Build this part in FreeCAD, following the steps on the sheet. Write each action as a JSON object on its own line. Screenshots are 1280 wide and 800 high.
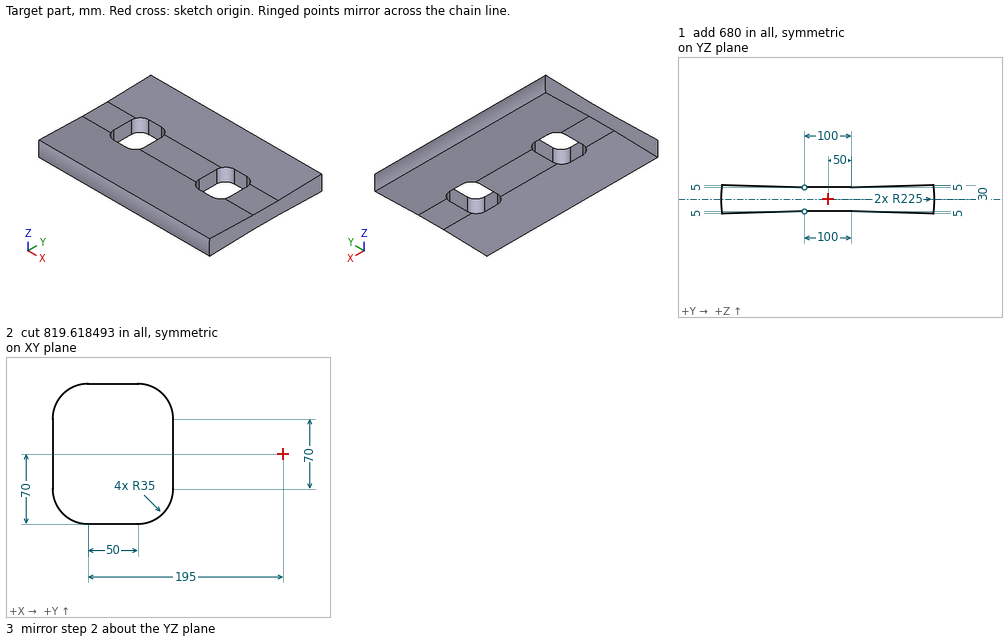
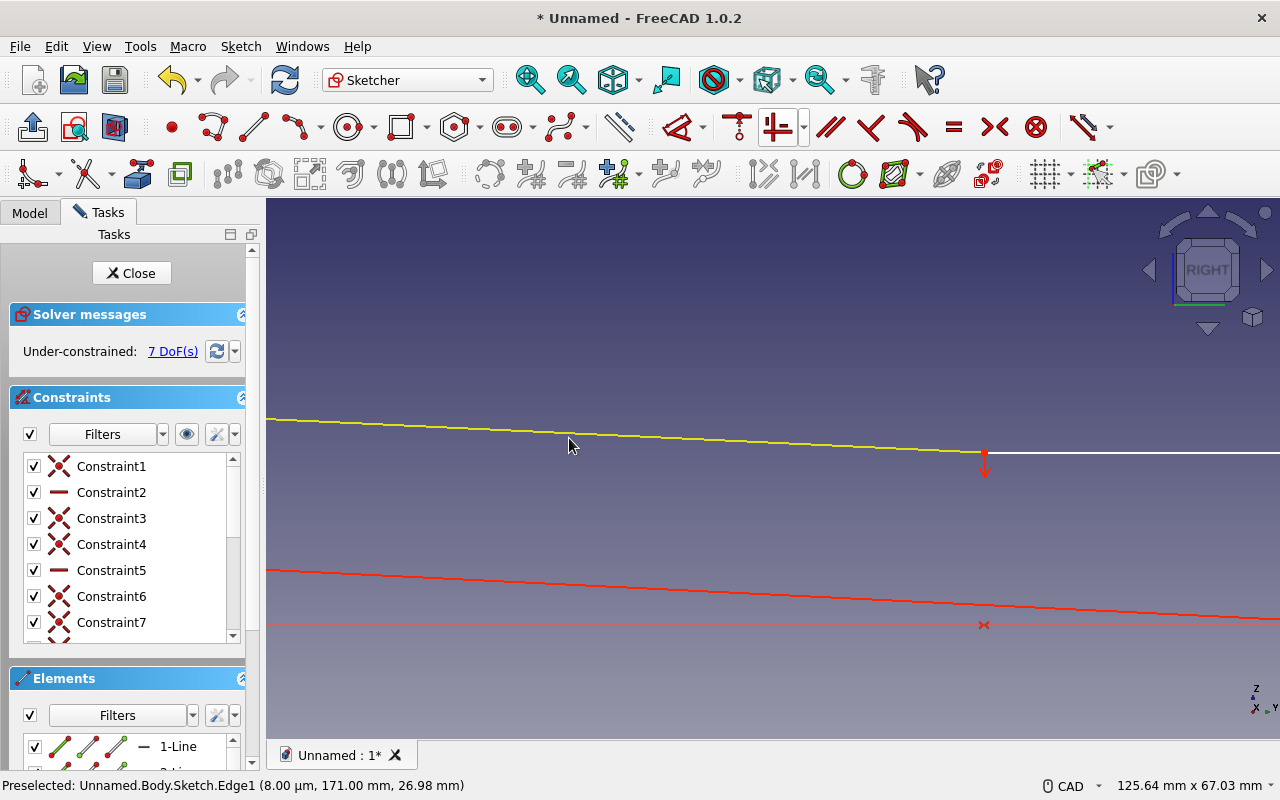
{"action": "left_click", "coordinate": [566, 433]}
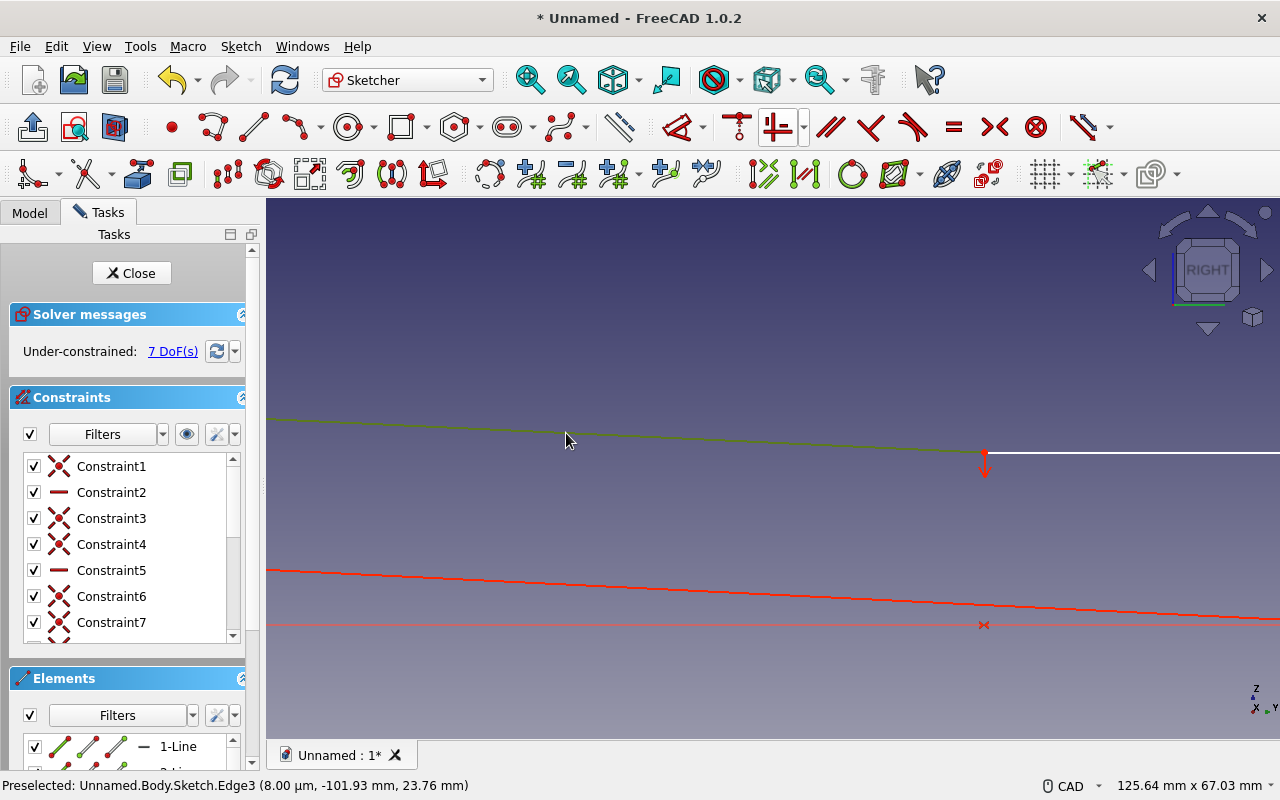
{"action": "key", "text": "i"}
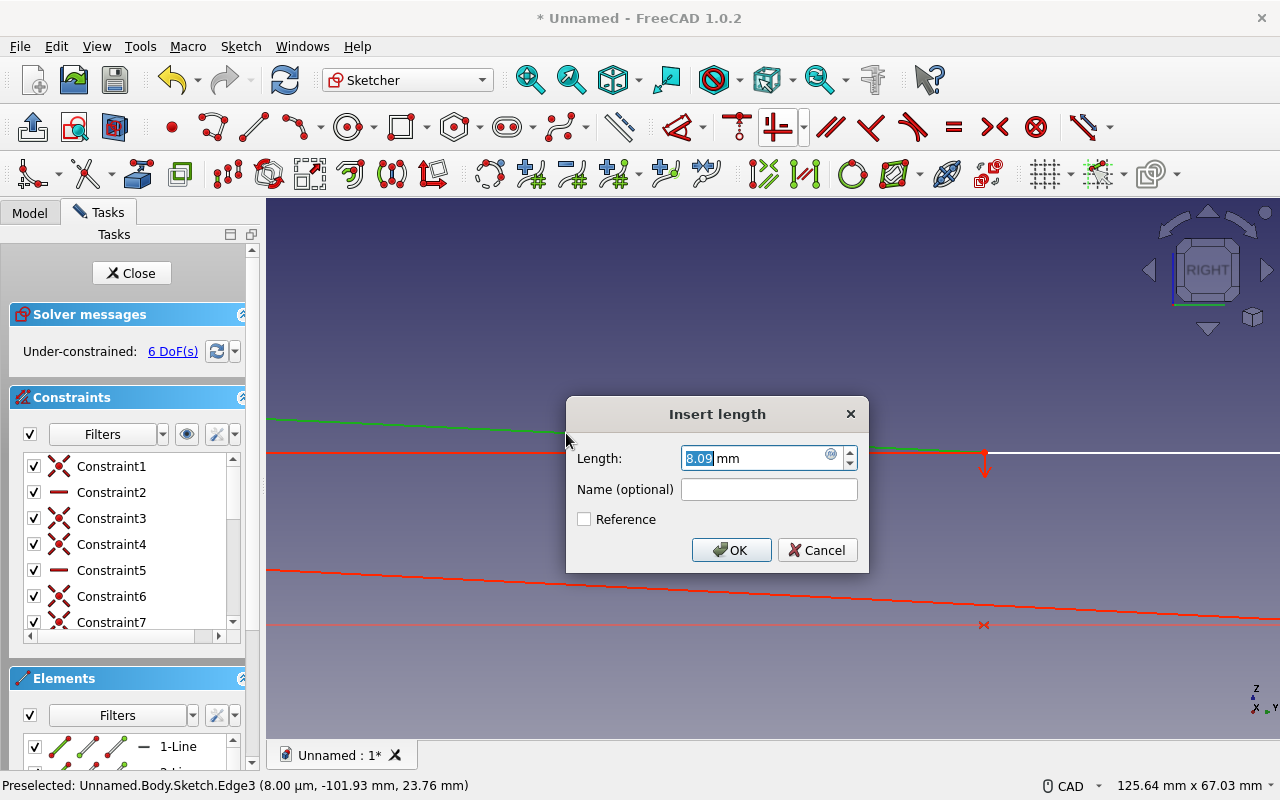
{"action": "type", "text": "5"}
{"action": "key", "text": "Return"}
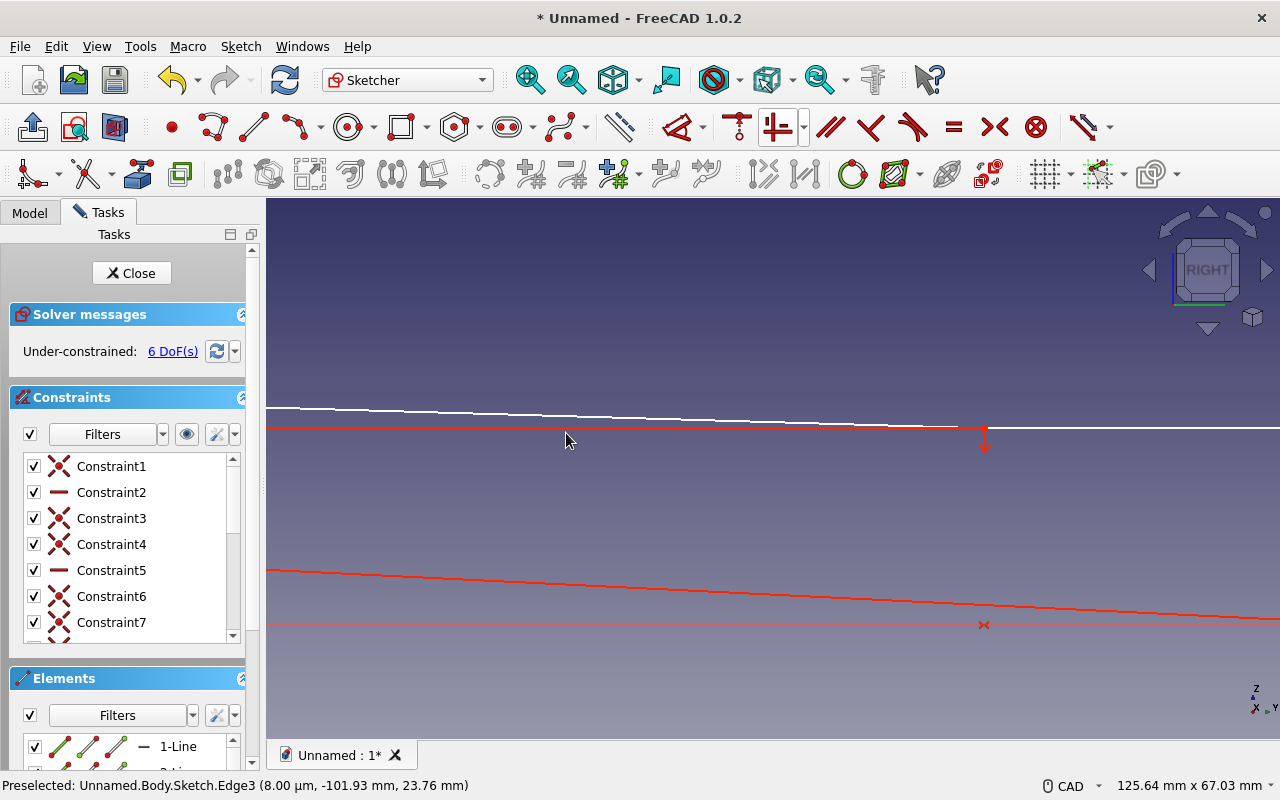
{"action": "scroll", "coordinate": [569, 438], "scroll_direction": "down", "scroll_amount": 9}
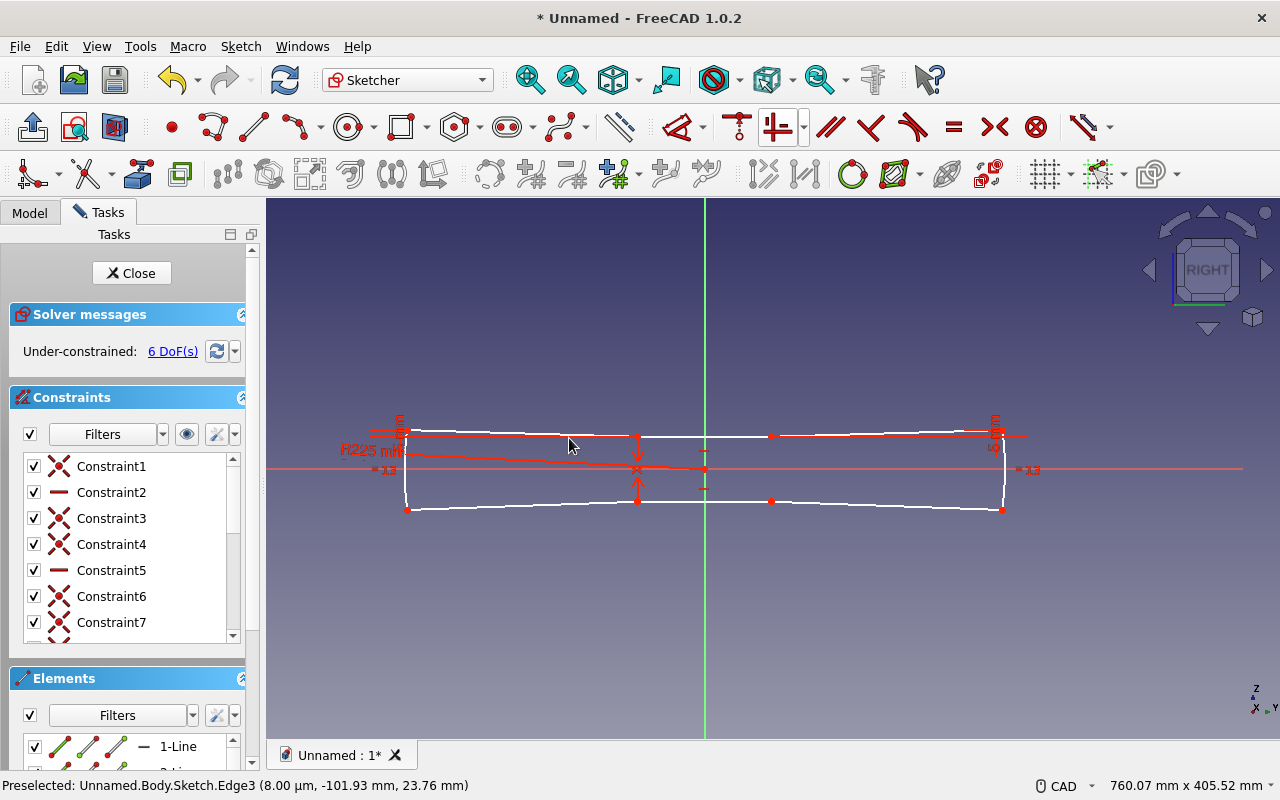
{"action": "scroll", "coordinate": [477, 508], "scroll_direction": "up", "scroll_amount": 9}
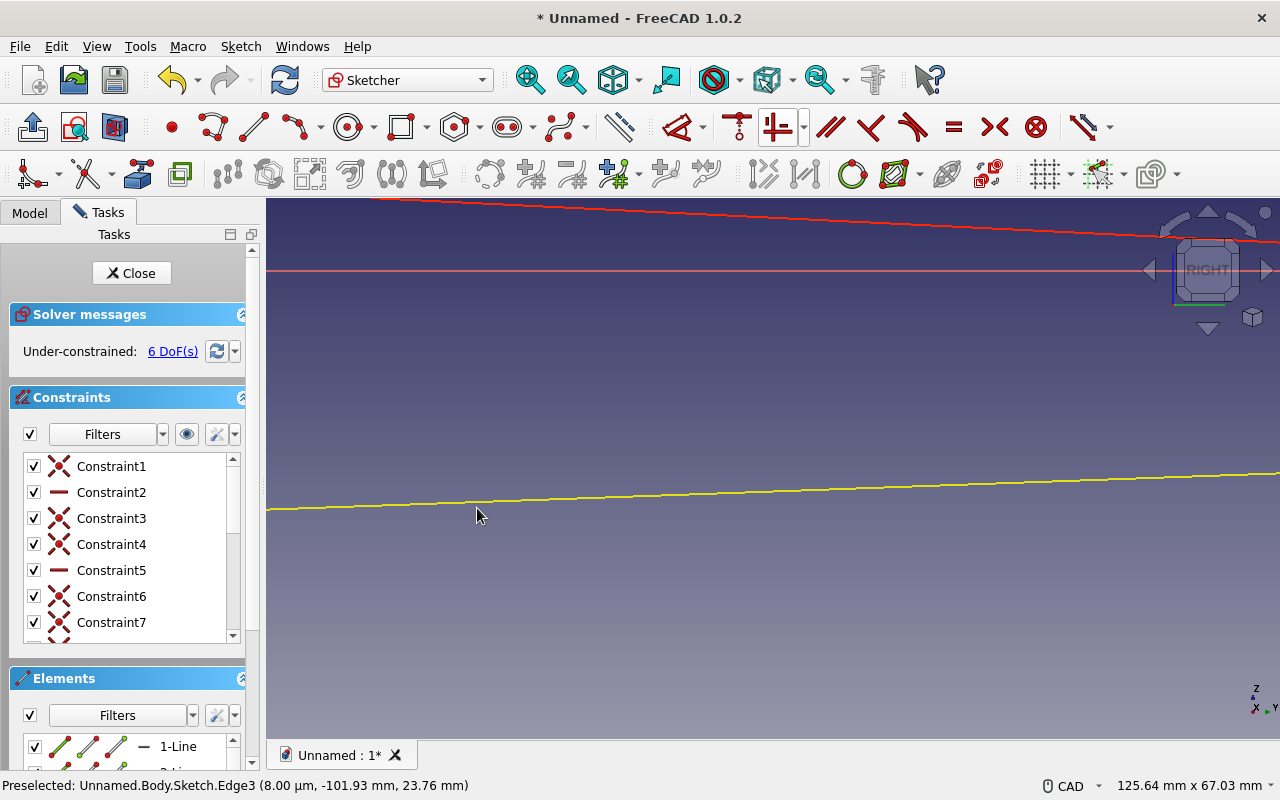
{"action": "left_click", "coordinate": [473, 502]}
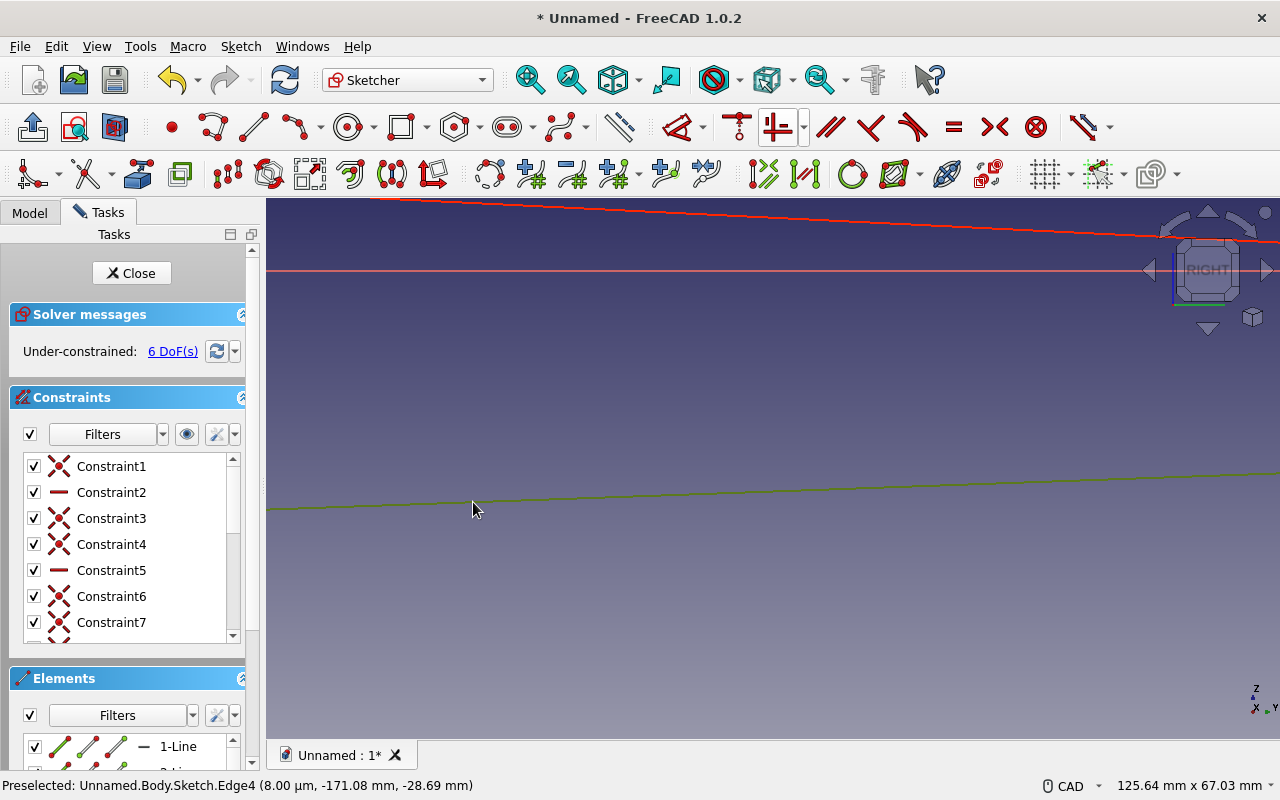
{"action": "key", "text": "i"}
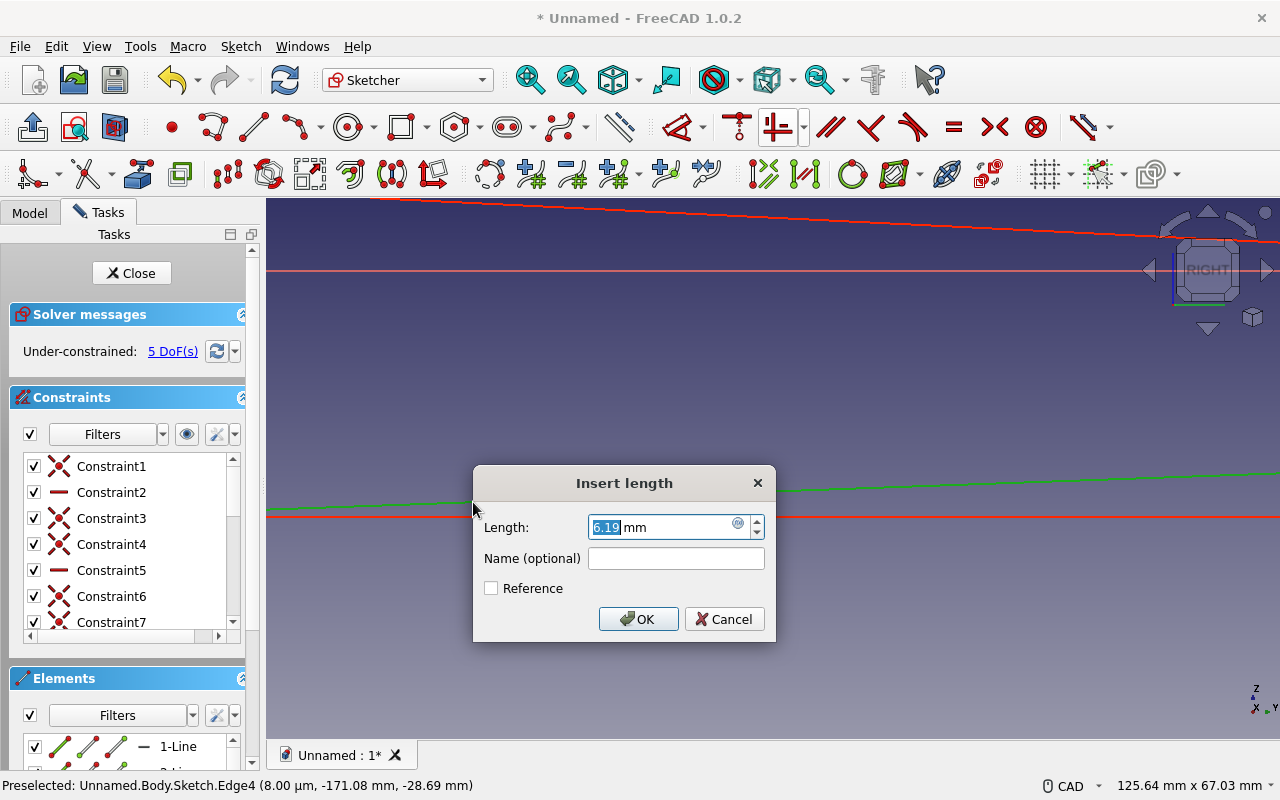
{"action": "type", "text": "5"}
{"action": "key", "text": "Return"}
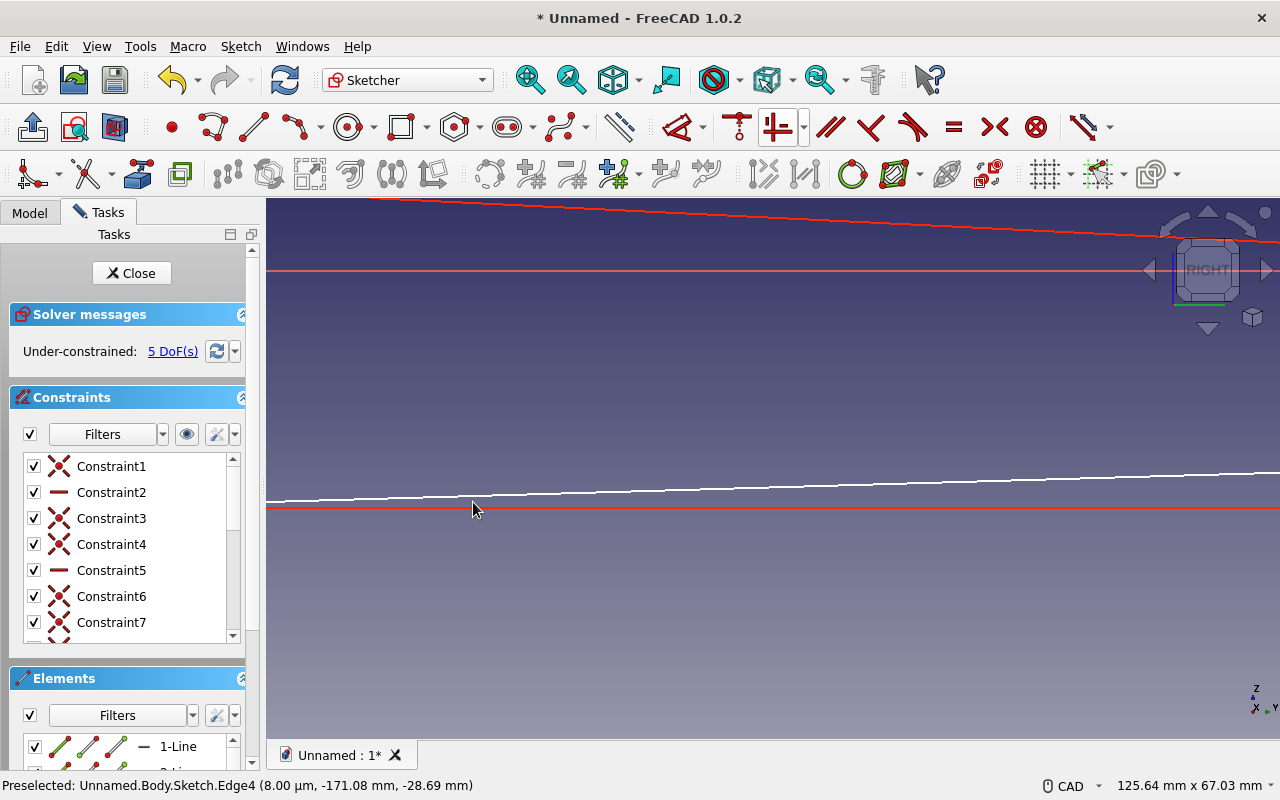
{"action": "scroll", "coordinate": [477, 508], "scroll_direction": "down", "scroll_amount": 9}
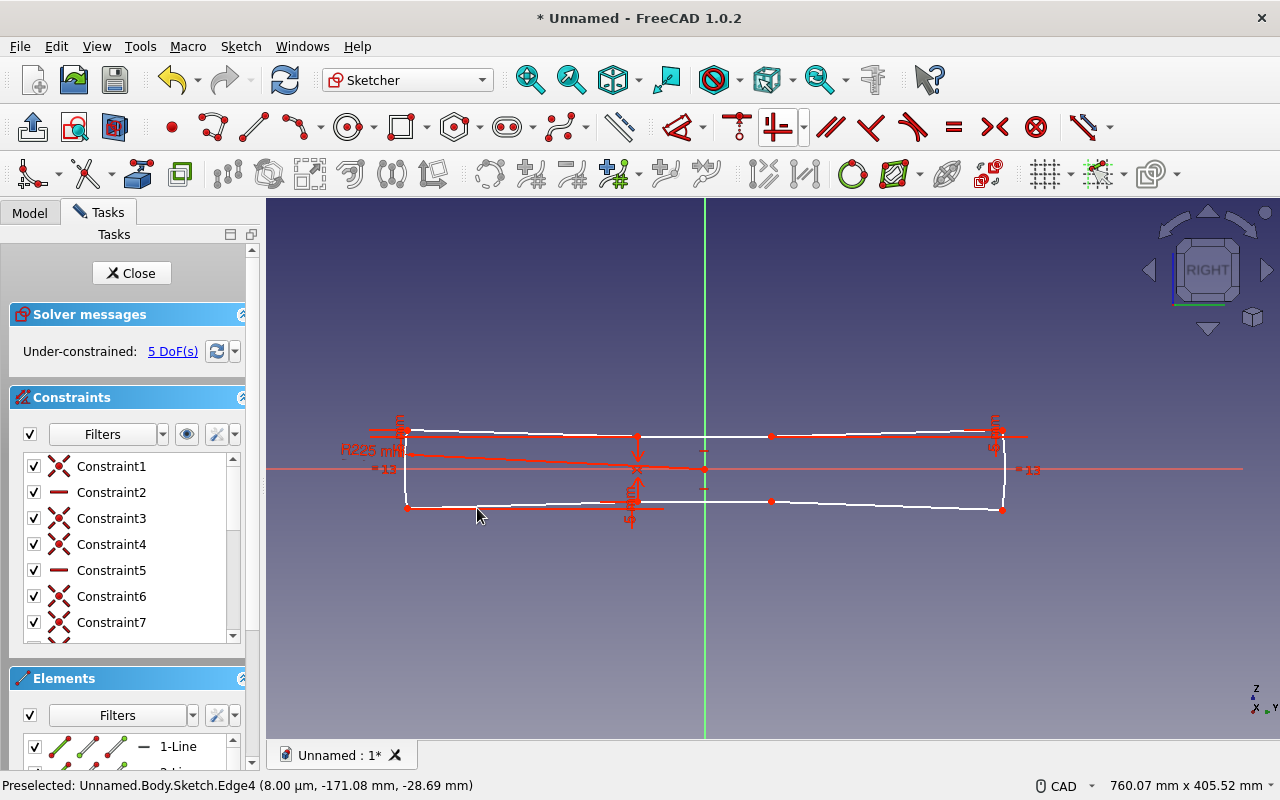
{"action": "scroll", "coordinate": [840, 504], "scroll_direction": "up", "scroll_amount": 9}